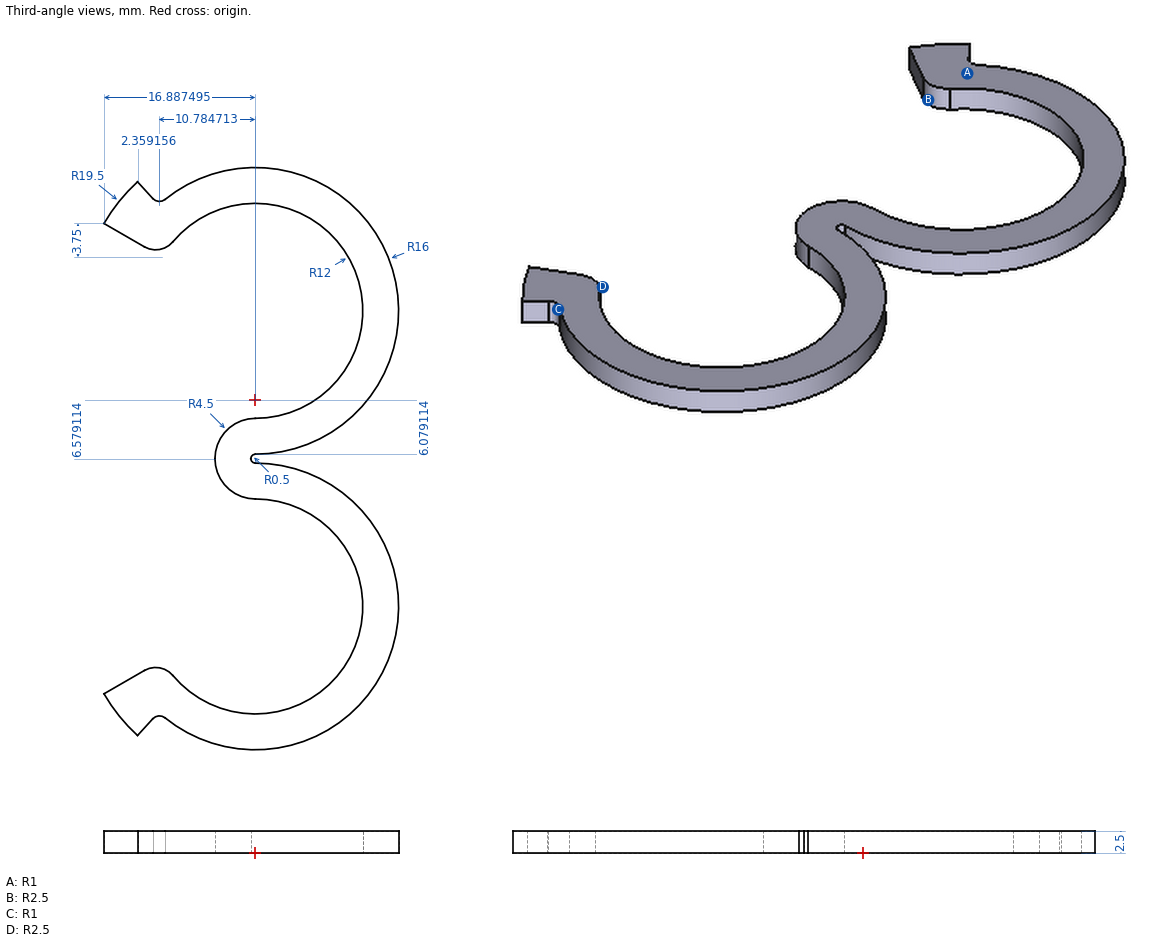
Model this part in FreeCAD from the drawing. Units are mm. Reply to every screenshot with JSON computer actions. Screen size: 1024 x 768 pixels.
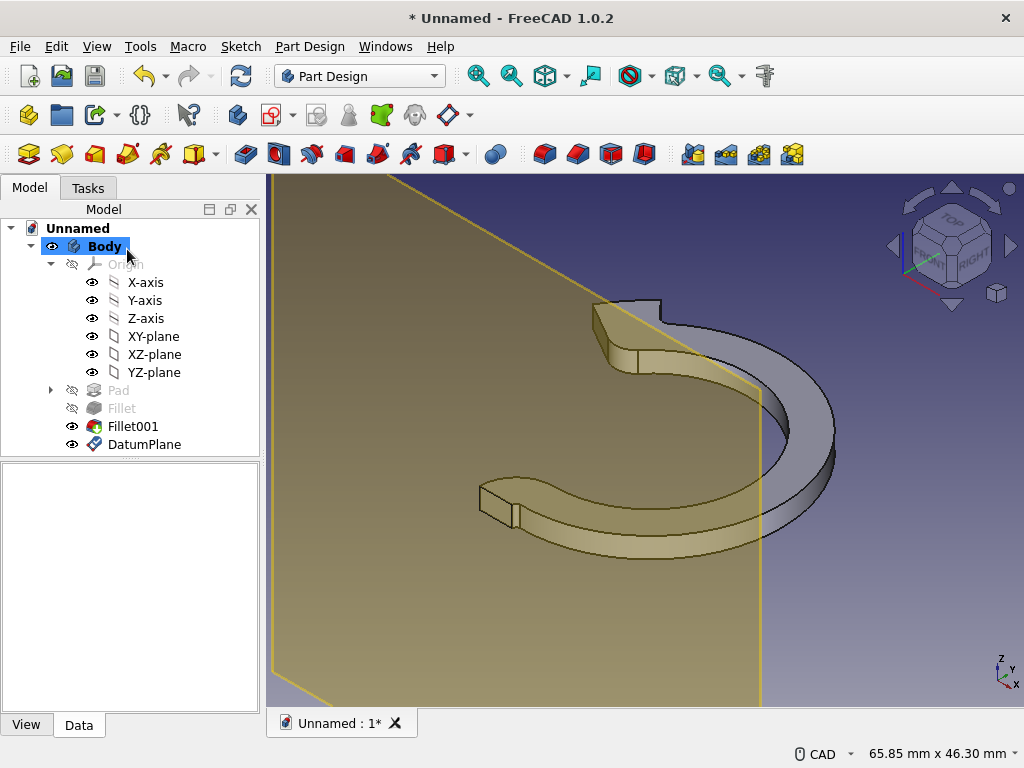
{"action": "left_click", "coordinate": [117, 390]}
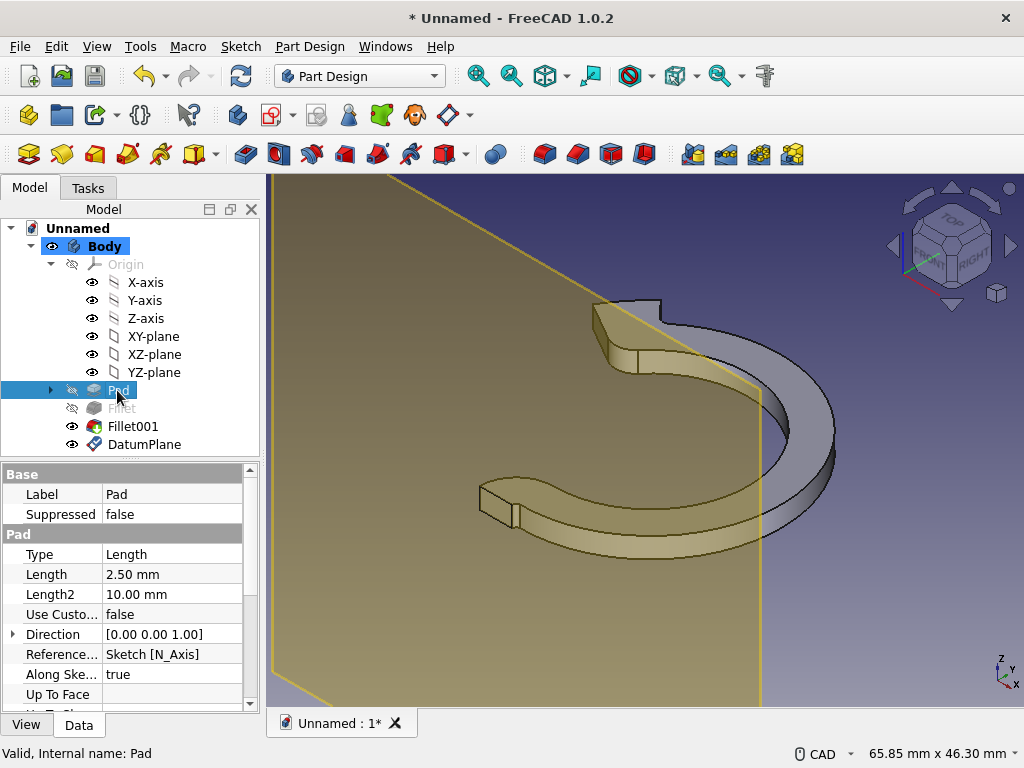
{"action": "left_click", "coordinate": [693, 154]}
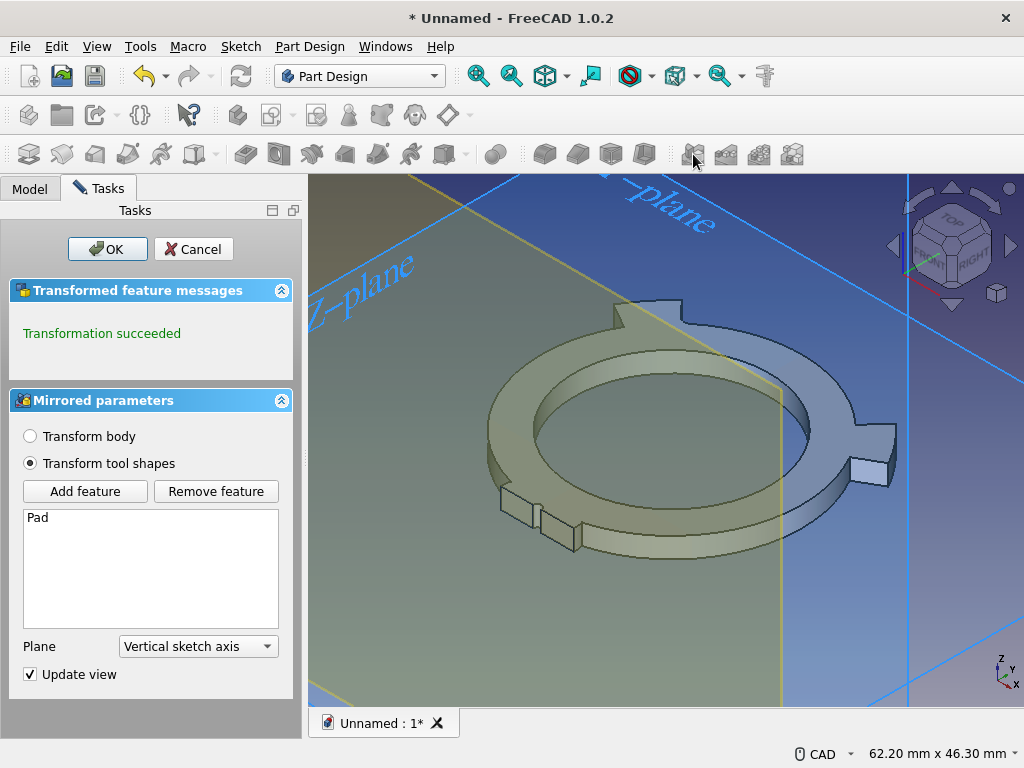
{"action": "left_click", "coordinate": [199, 646]}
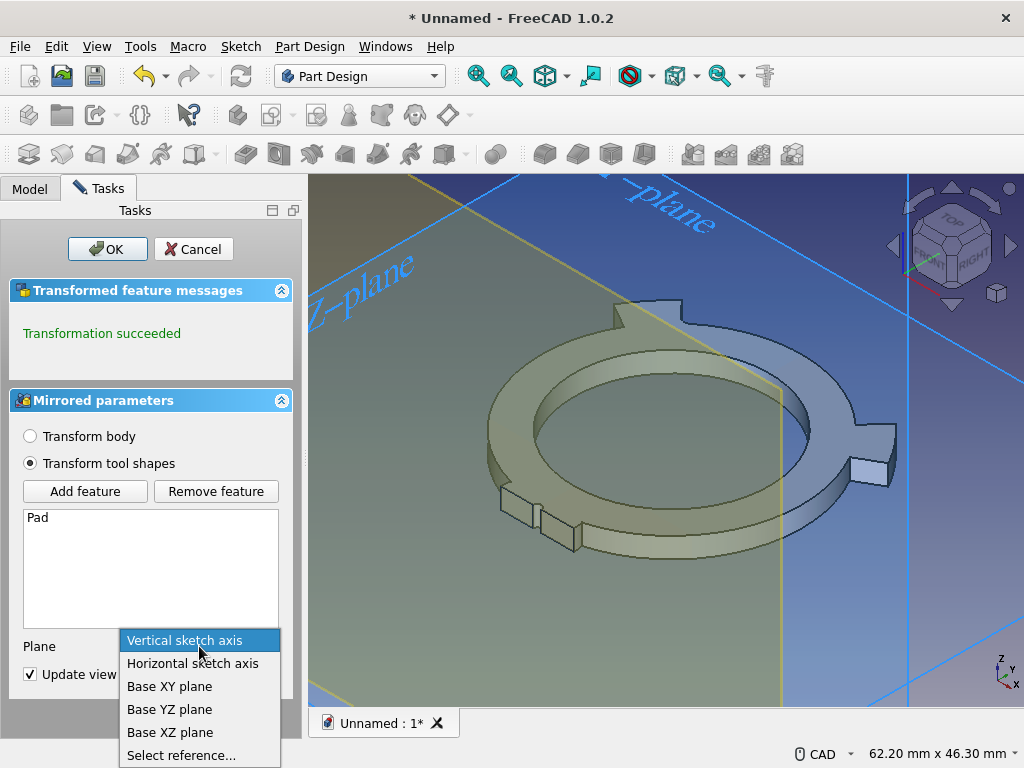
{"action": "left_click", "coordinate": [198, 756]}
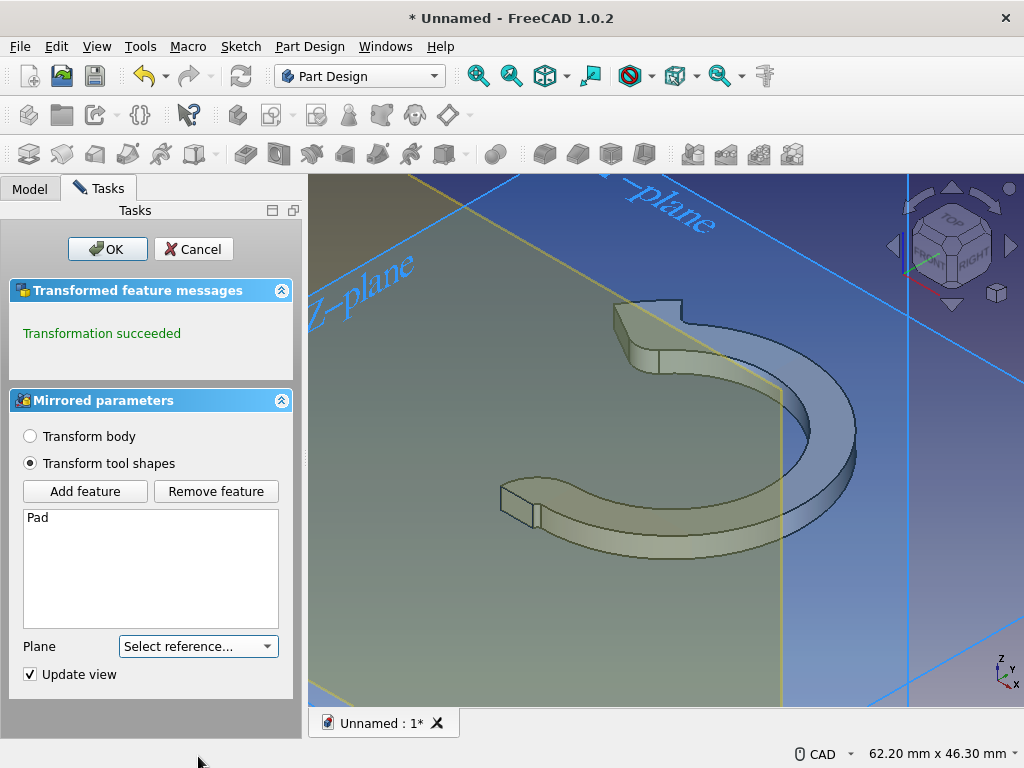
{"action": "left_click", "coordinate": [30, 188]}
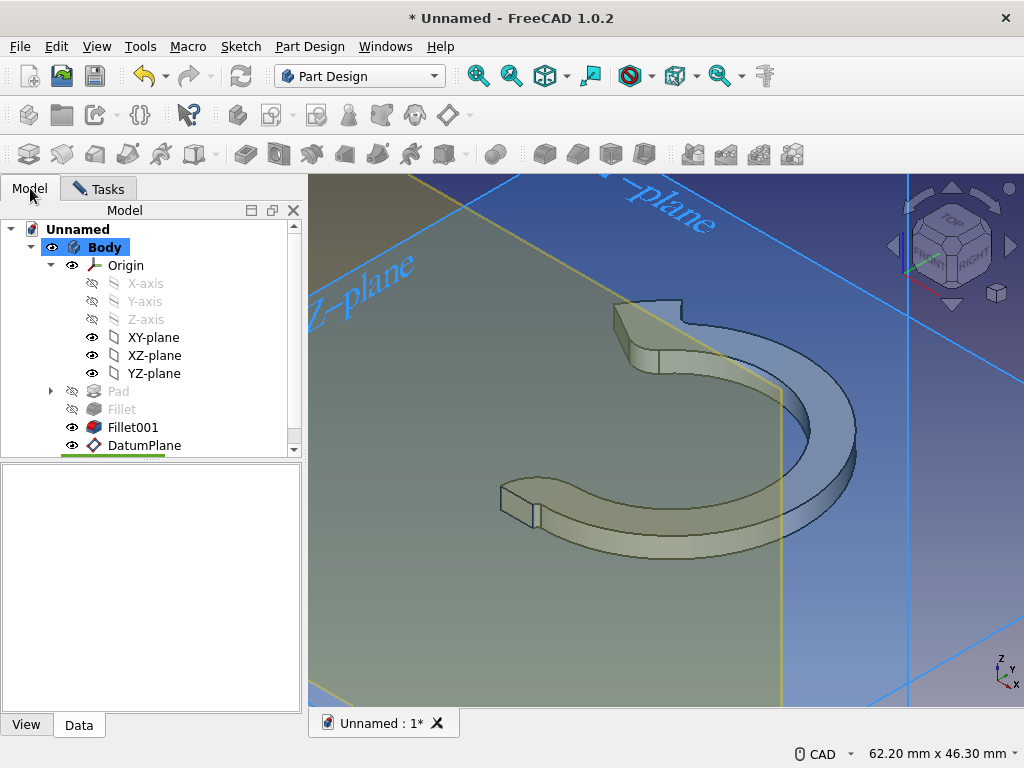
{"action": "left_click", "coordinate": [117, 445]}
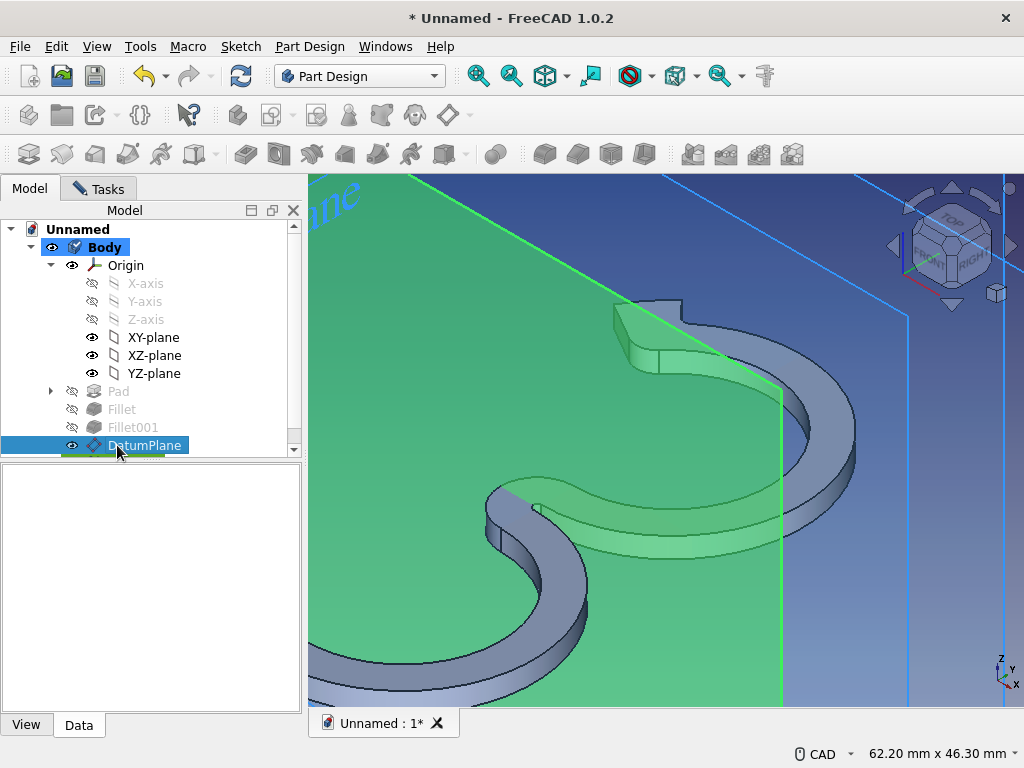
{"action": "left_click", "coordinate": [98, 188]}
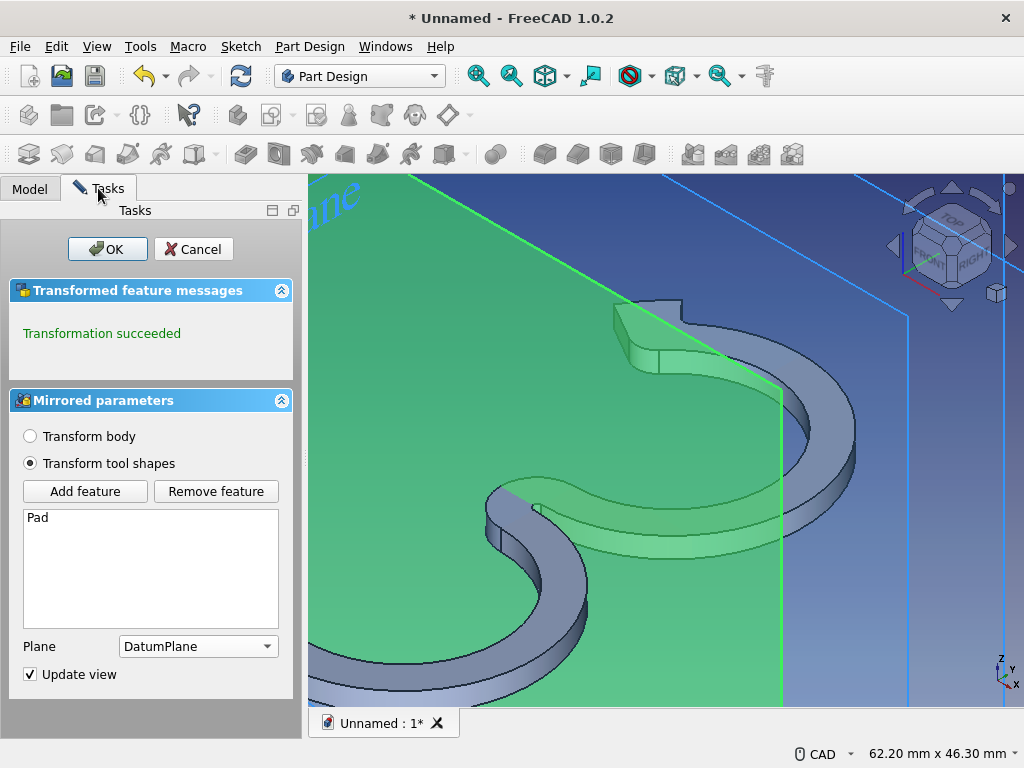
{"action": "left_click", "coordinate": [108, 249]}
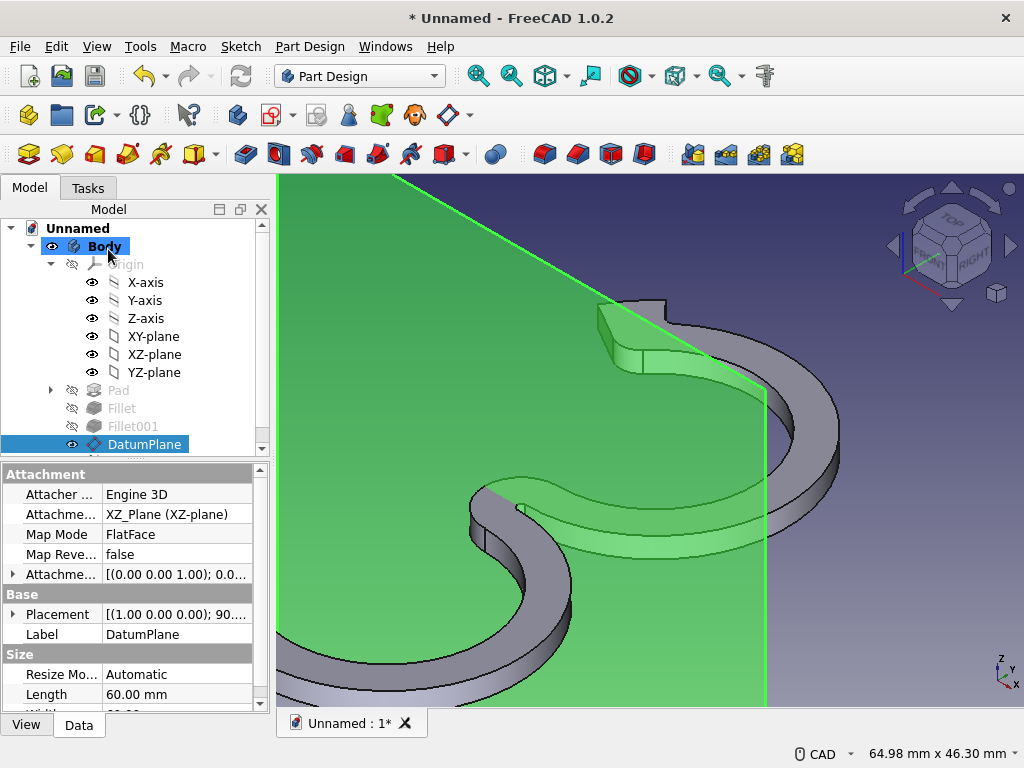
{"action": "left_click", "coordinate": [117, 444]}
{"action": "key", "text": "space"}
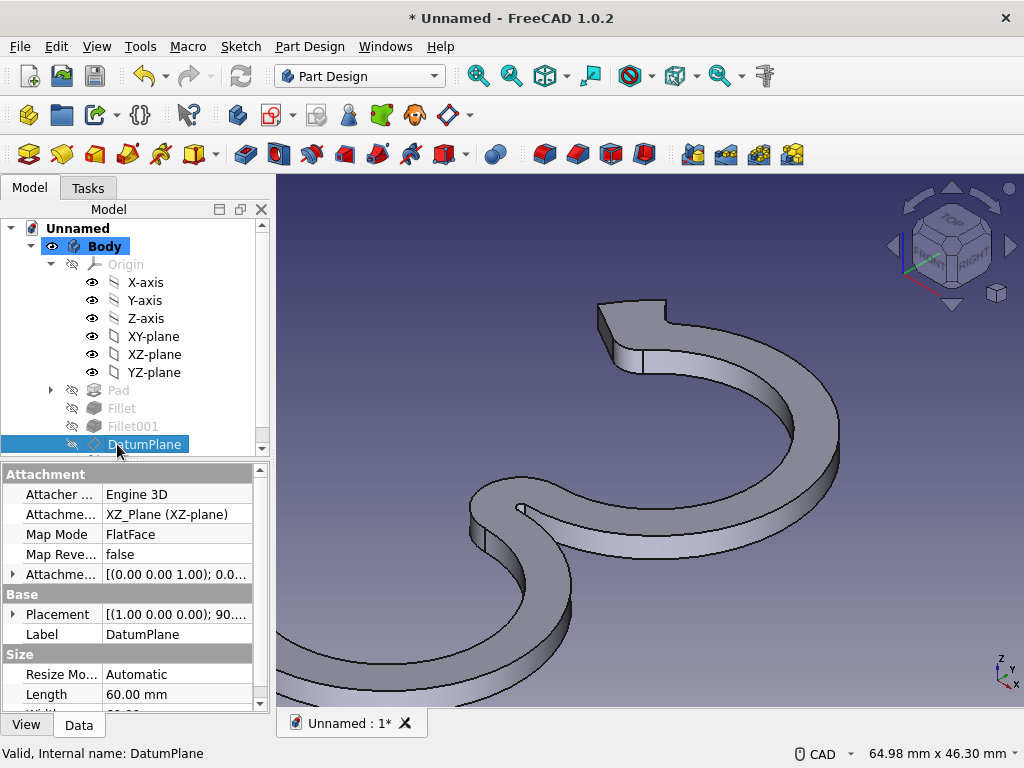
{"action": "left_click", "coordinate": [479, 76]}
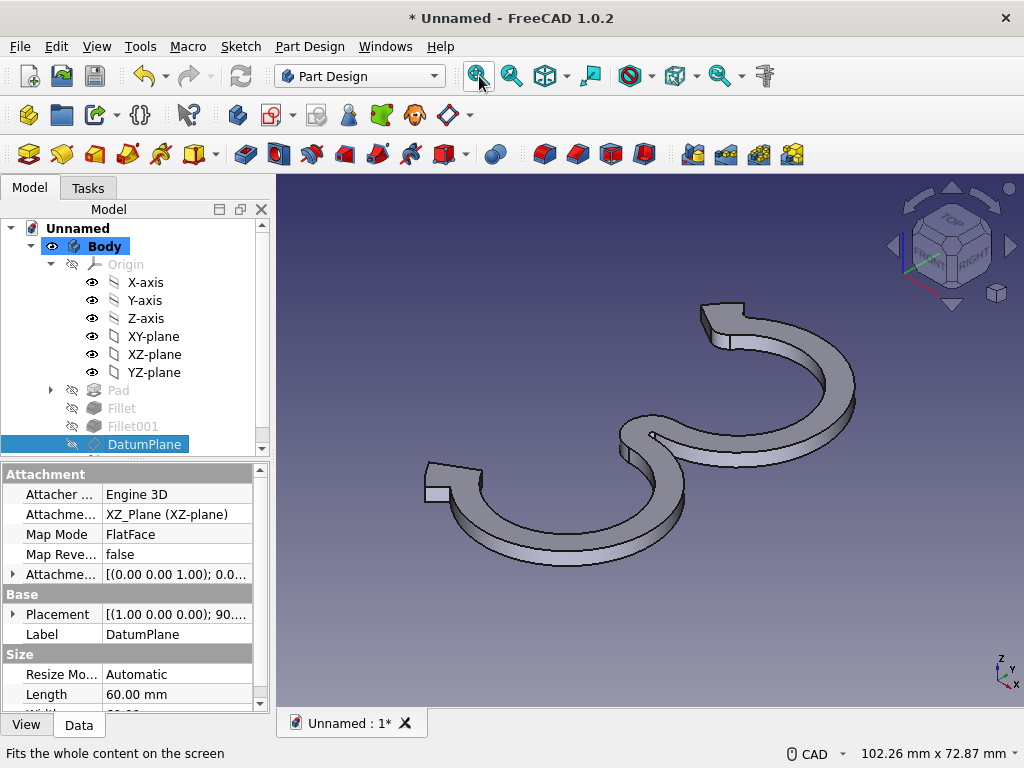
{"action": "scroll", "coordinate": [450, 493], "scroll_direction": "up", "scroll_amount": 4}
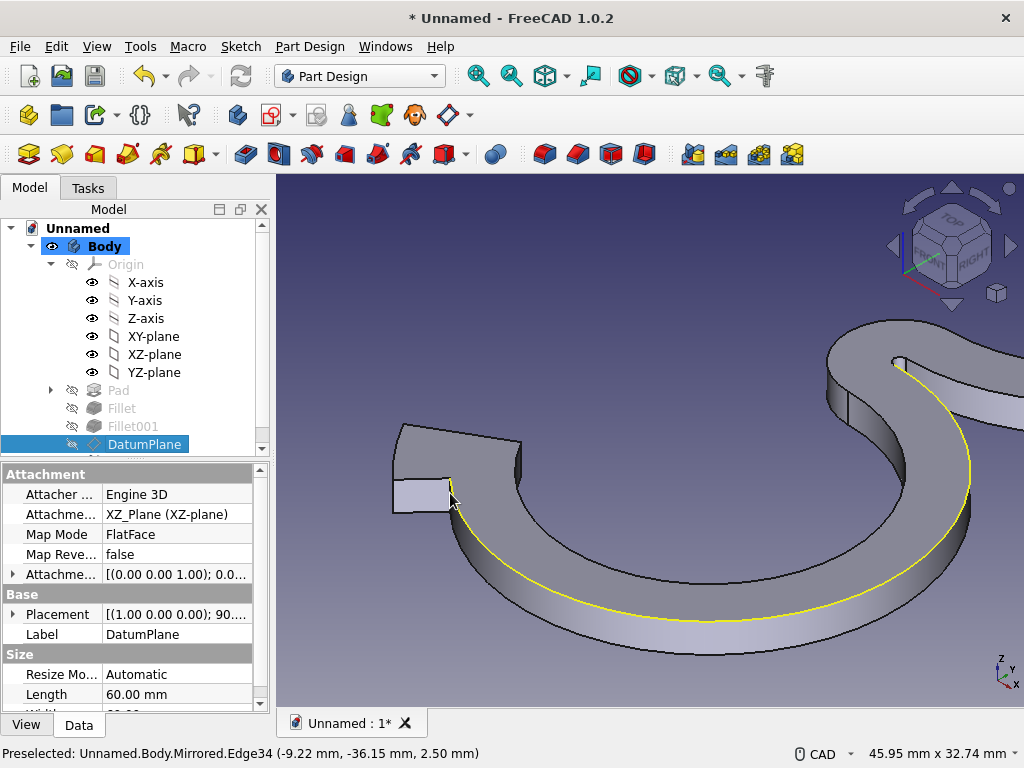
{"action": "left_click", "coordinate": [479, 76]}